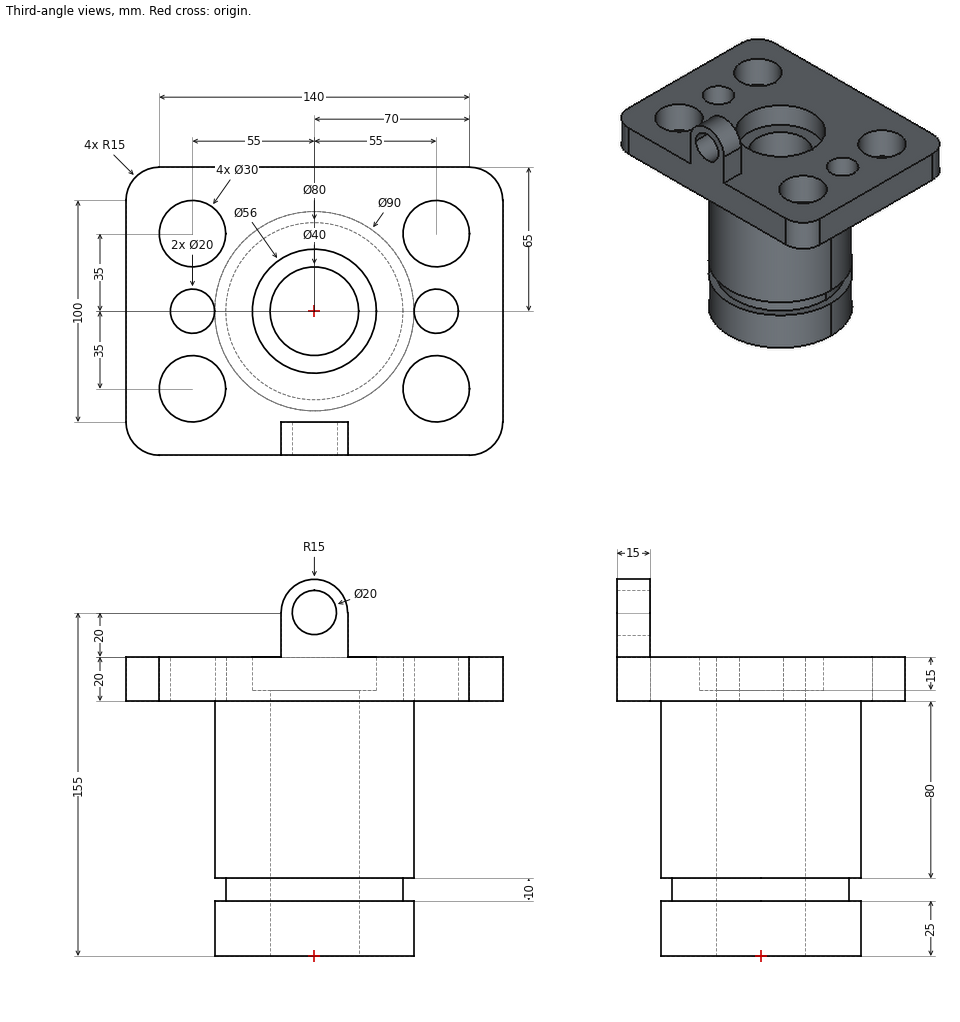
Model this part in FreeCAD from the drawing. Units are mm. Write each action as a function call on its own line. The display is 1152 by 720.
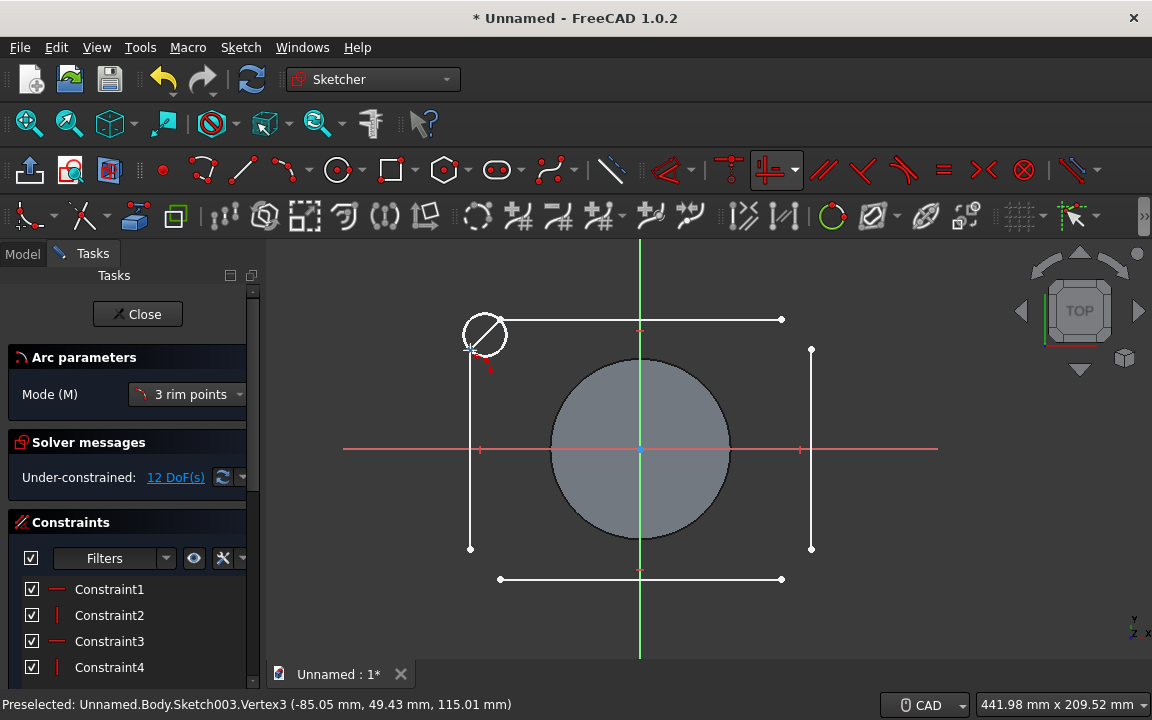
scroll(479, 328, up, 3)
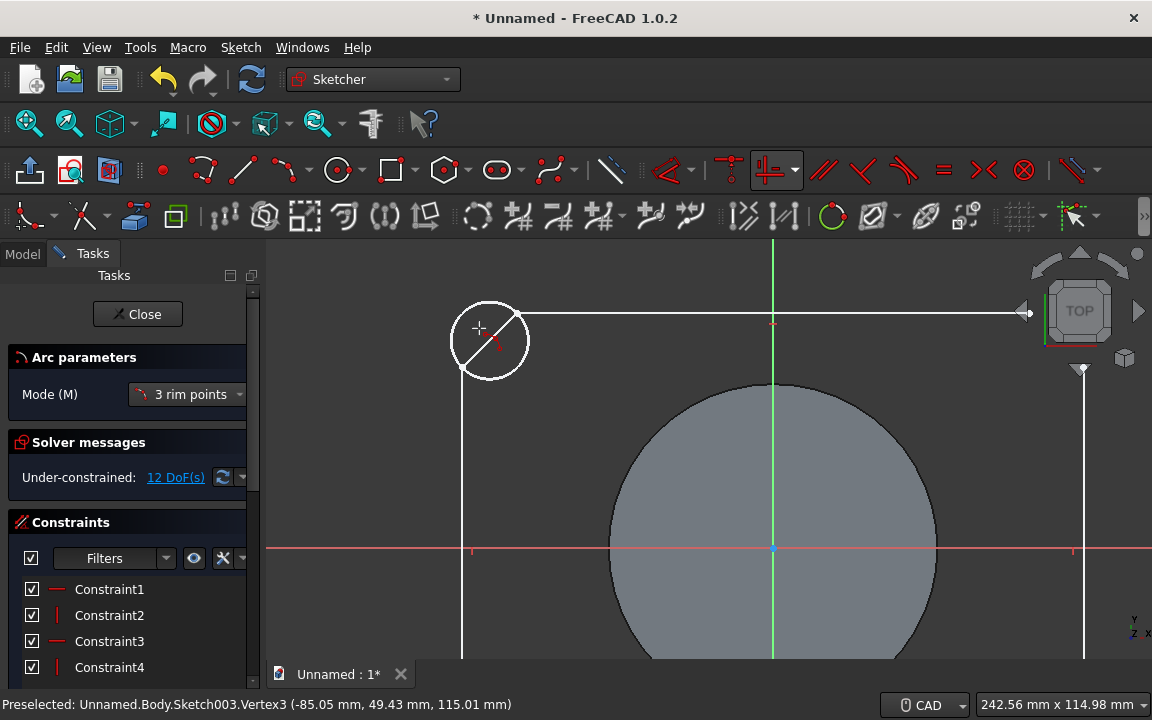
click(479, 327)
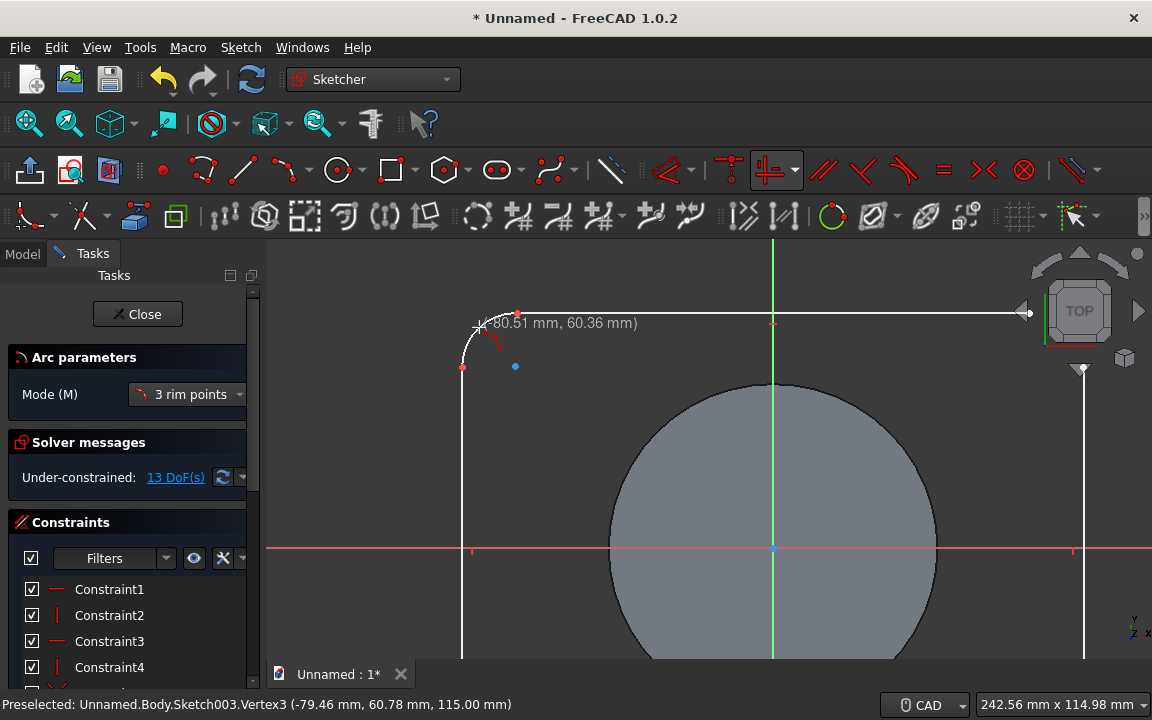
scroll(479, 328, down, 3)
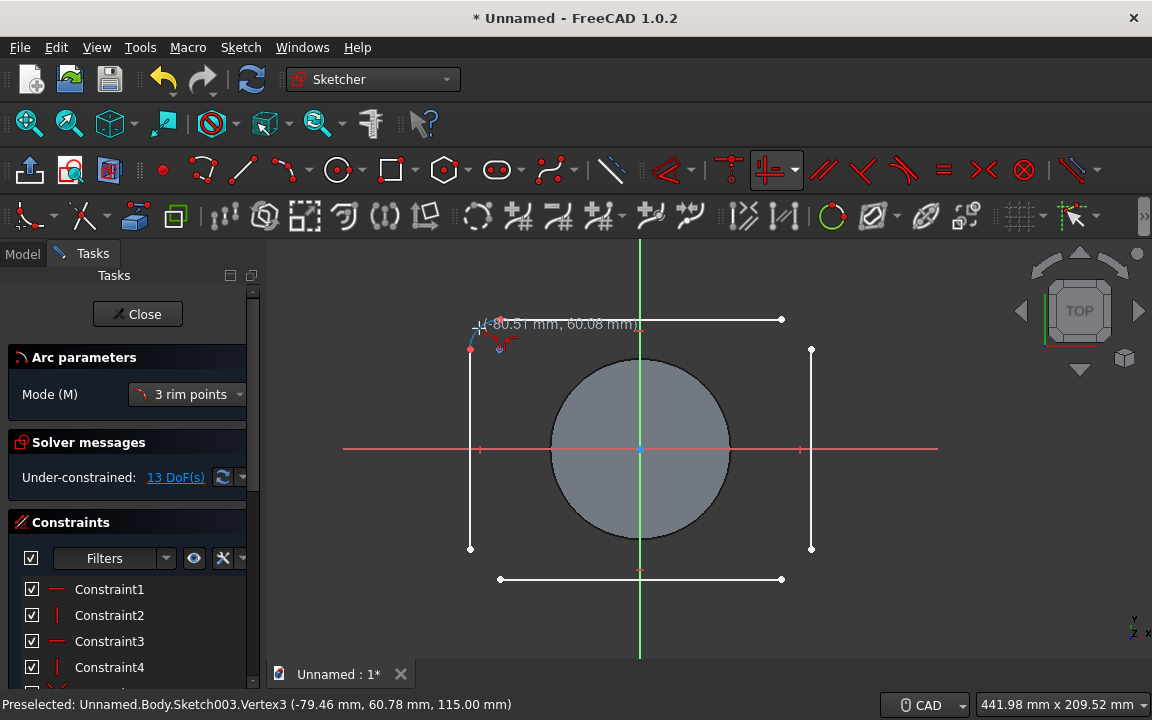
click(470, 550)
click(500, 580)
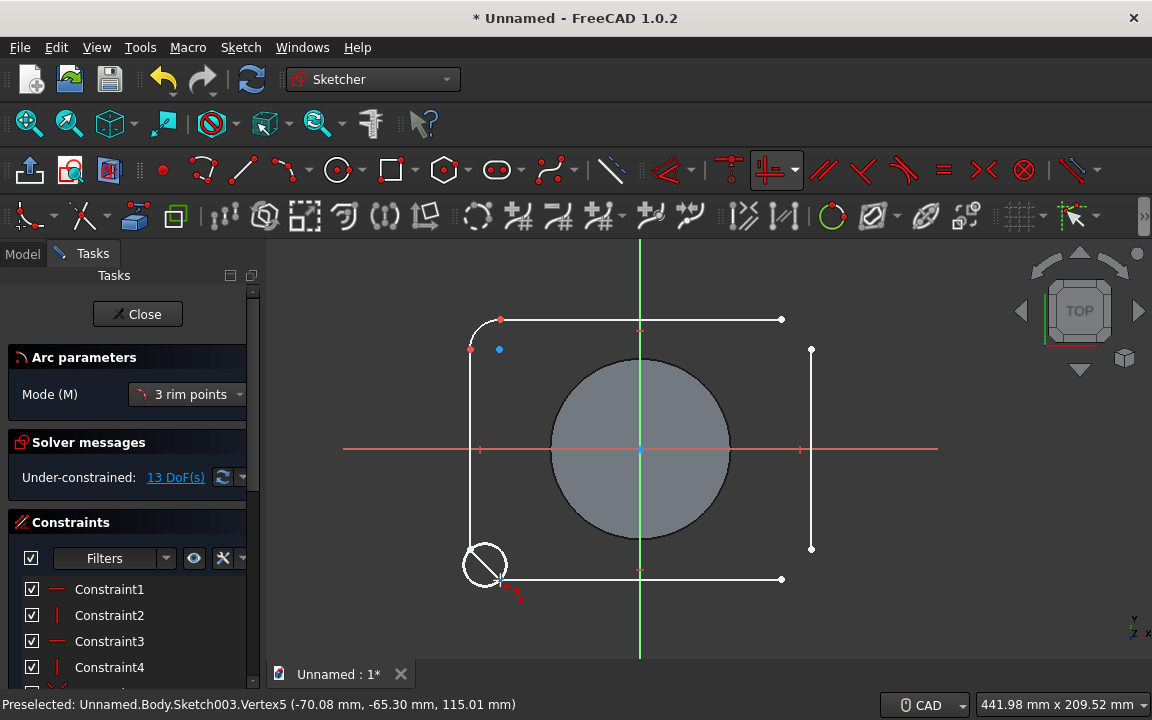
scroll(479, 571, up, 3)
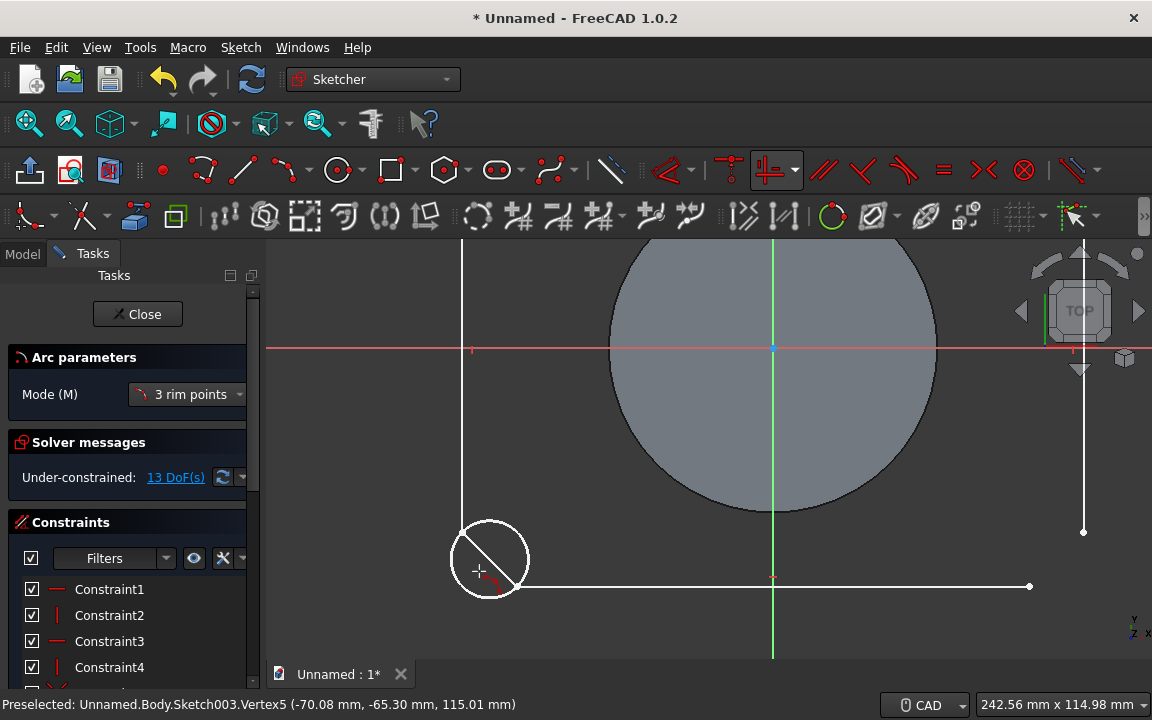
click(479, 570)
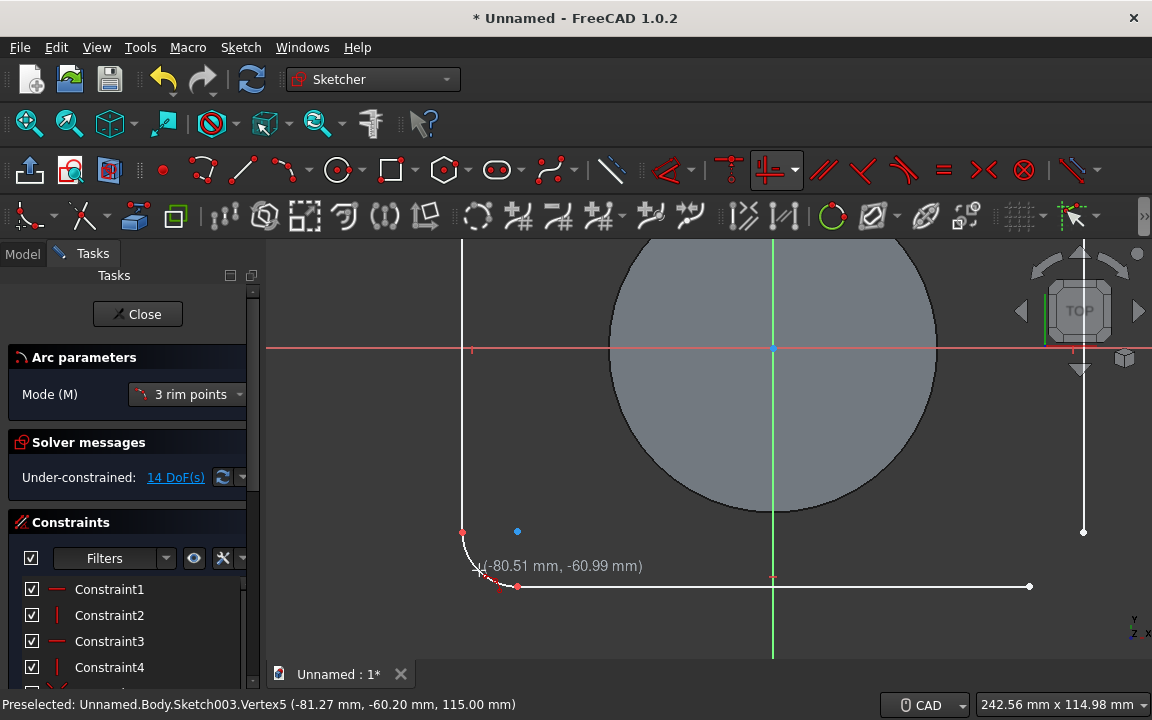
scroll(479, 572, down, 3)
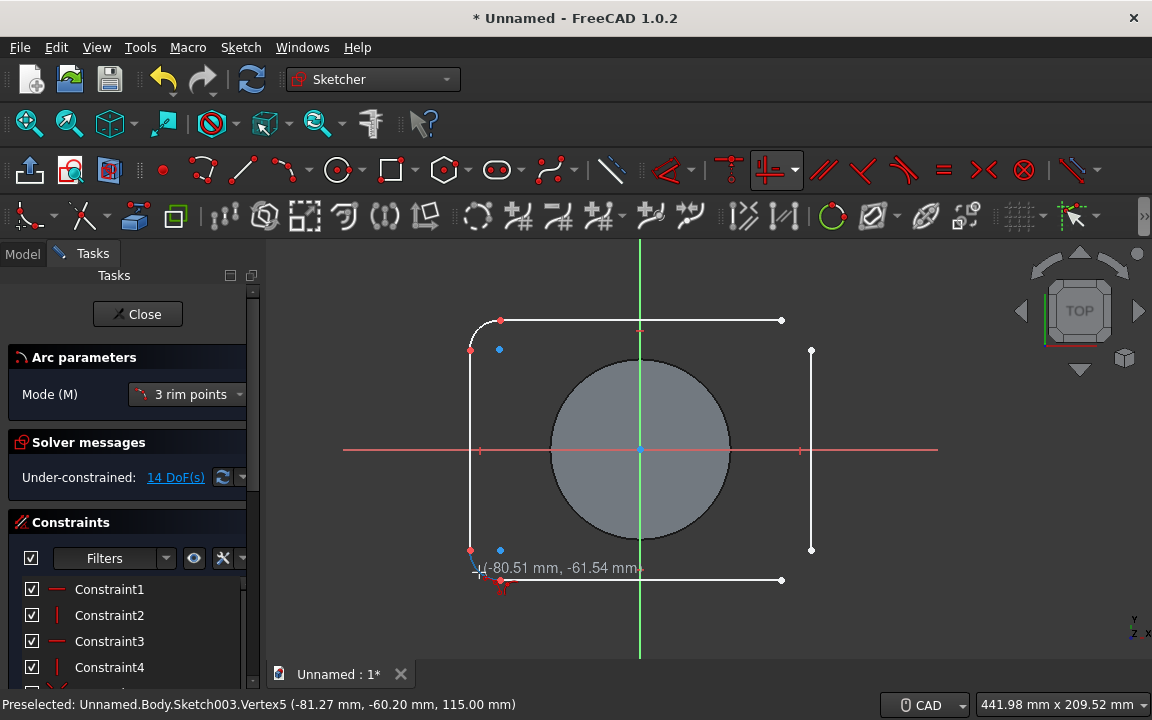
click(781, 580)
click(811, 550)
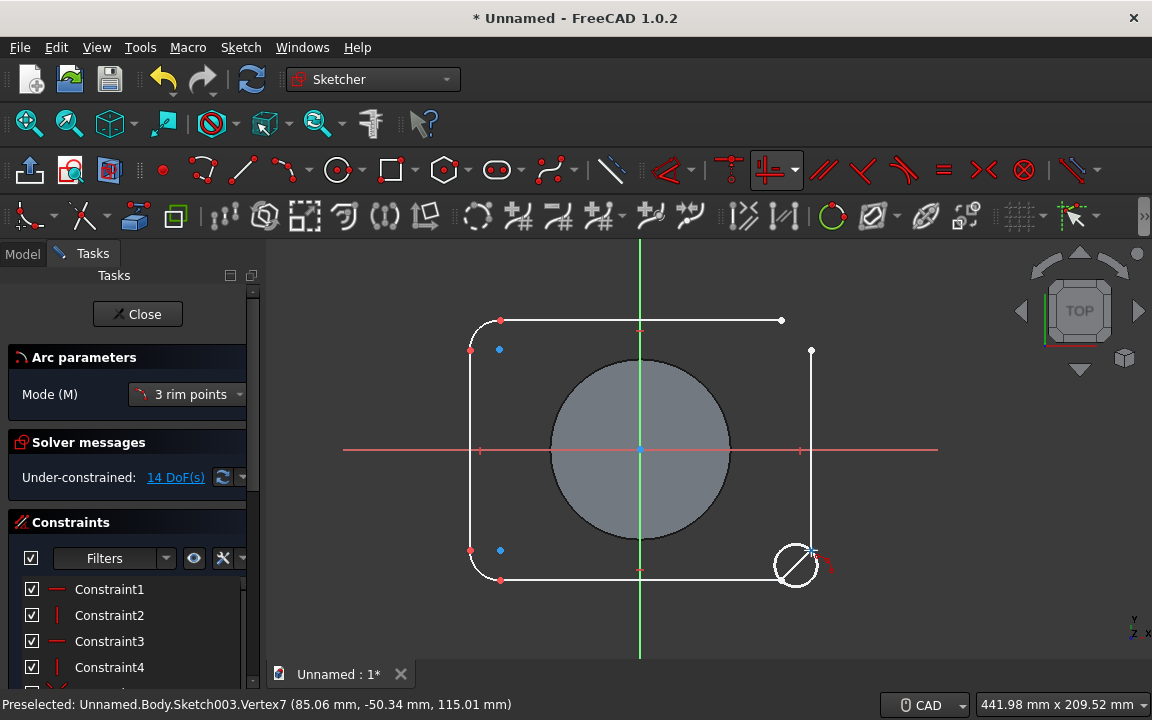
scroll(802, 571, up, 3)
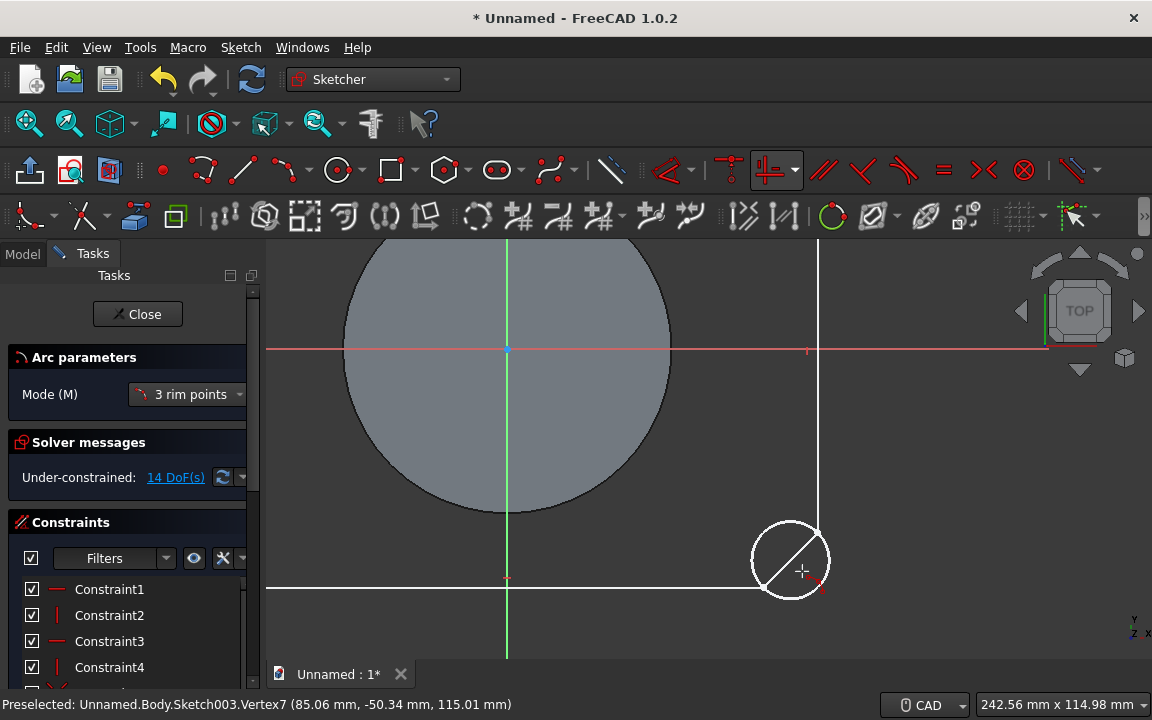
click(802, 570)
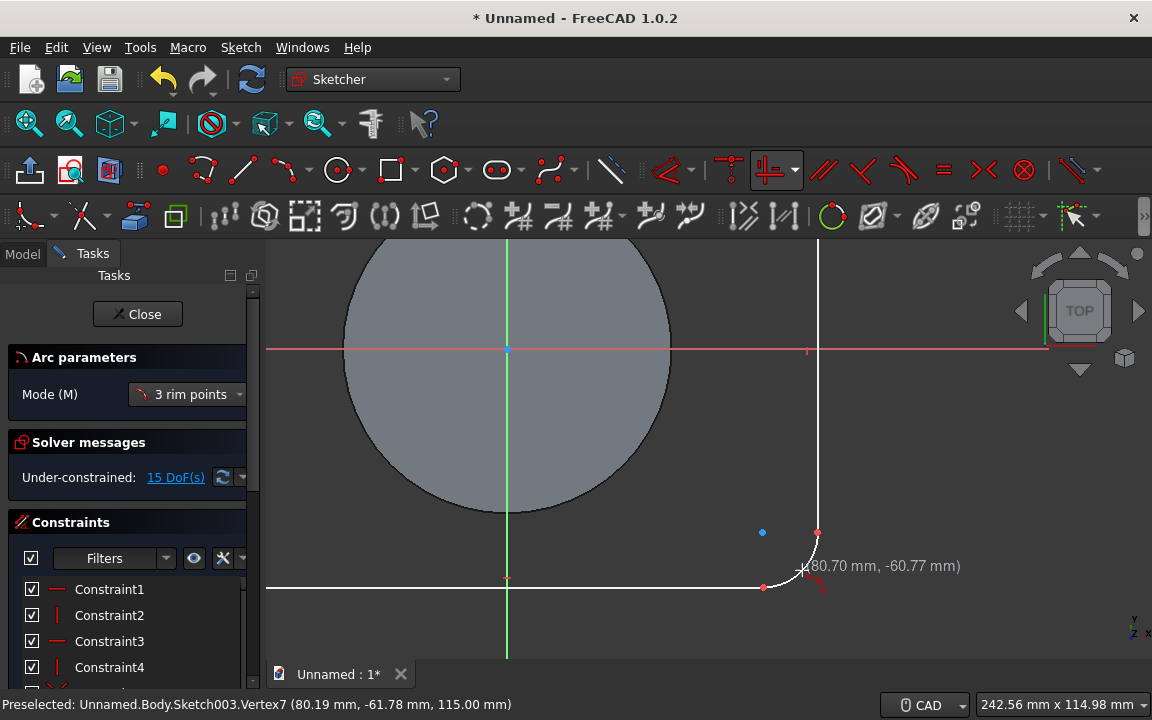
scroll(803, 571, down, 3)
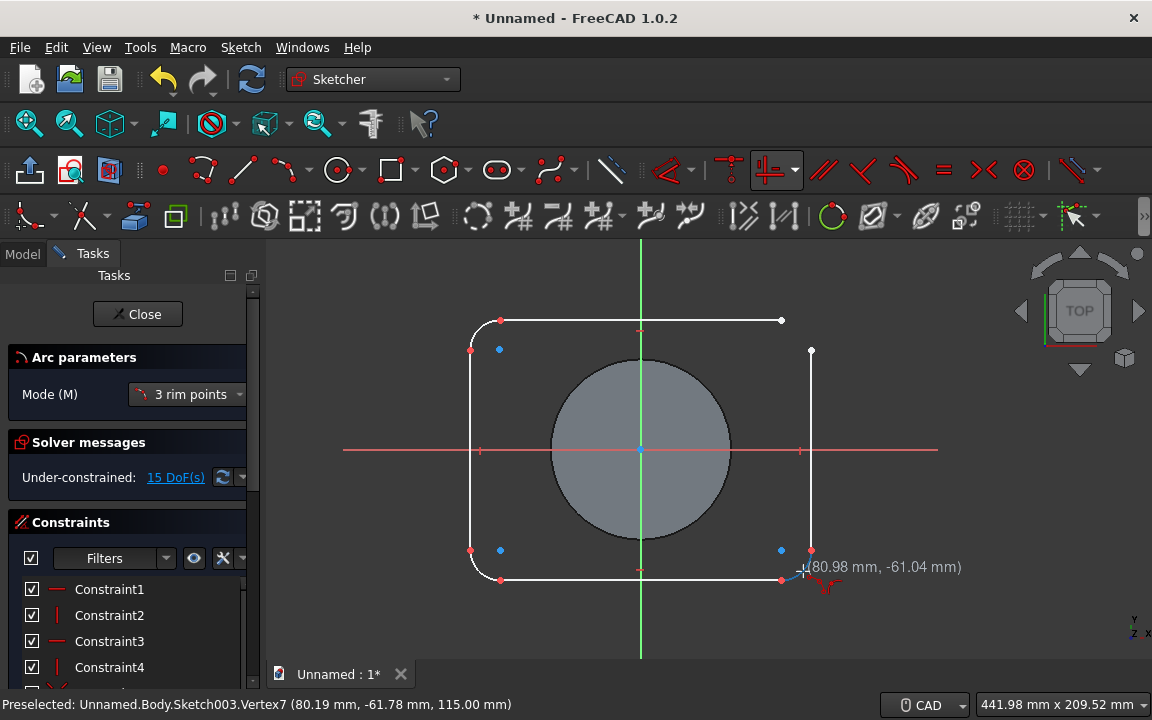
click(811, 350)
click(781, 320)